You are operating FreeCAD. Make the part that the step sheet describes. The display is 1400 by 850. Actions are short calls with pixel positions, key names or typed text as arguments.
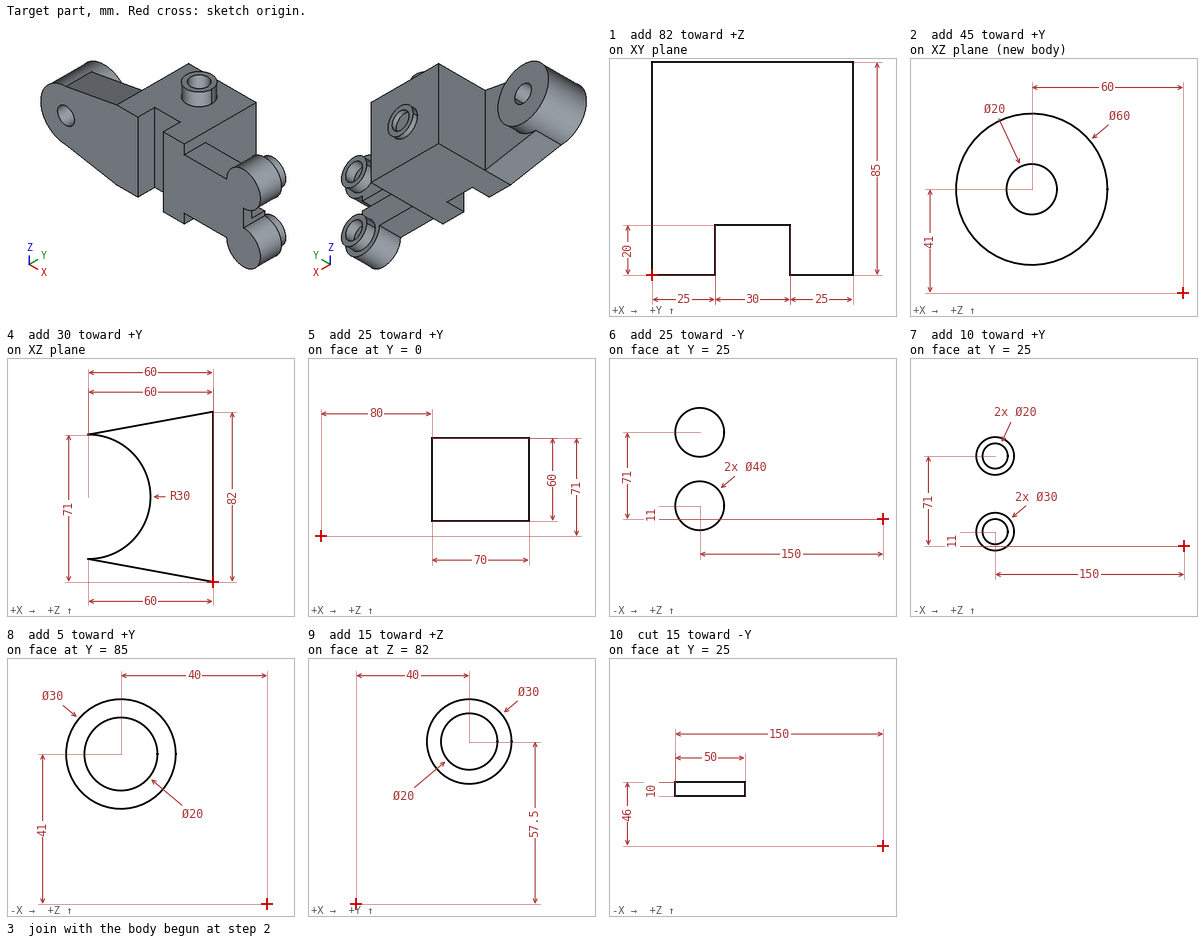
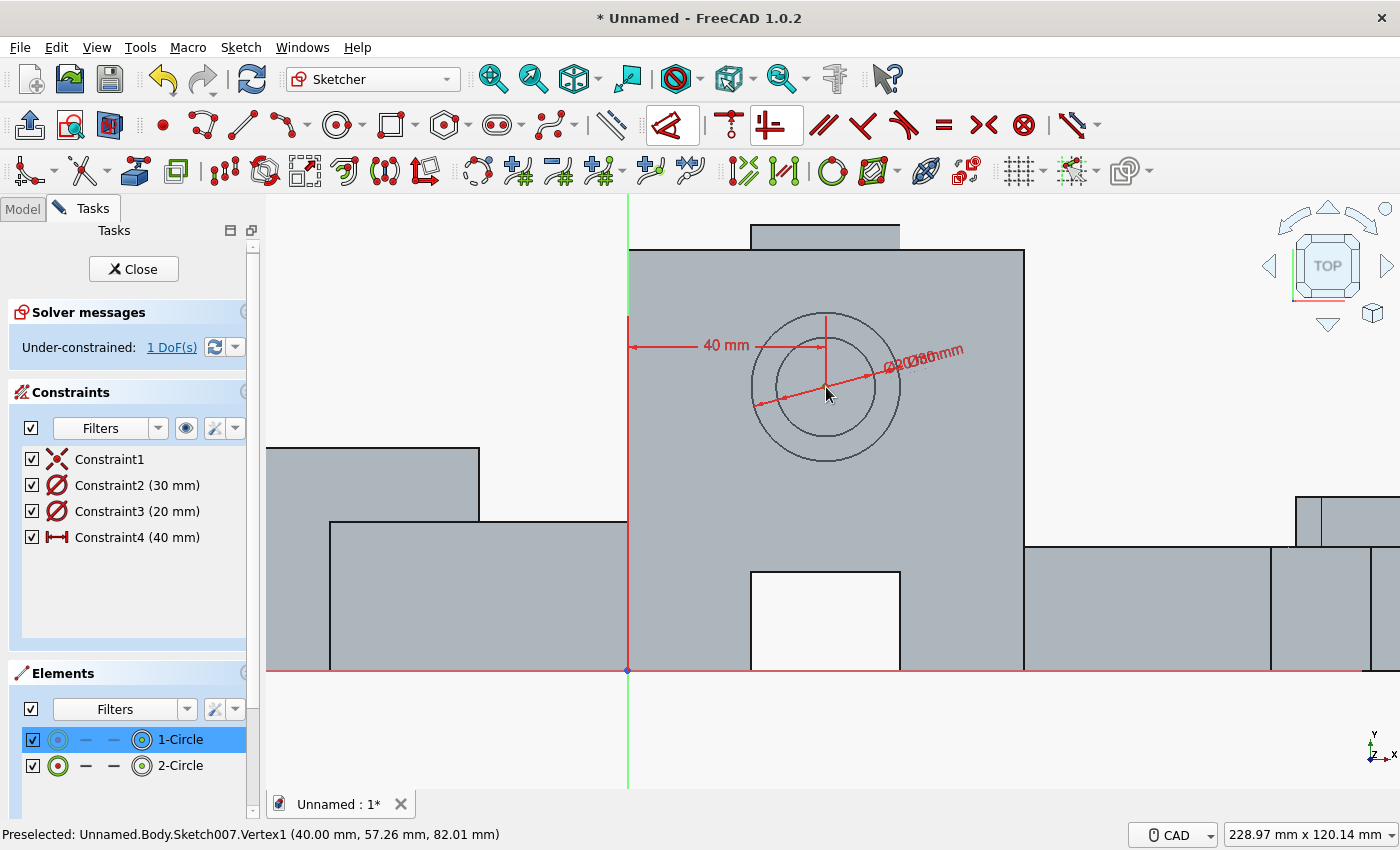
key(i)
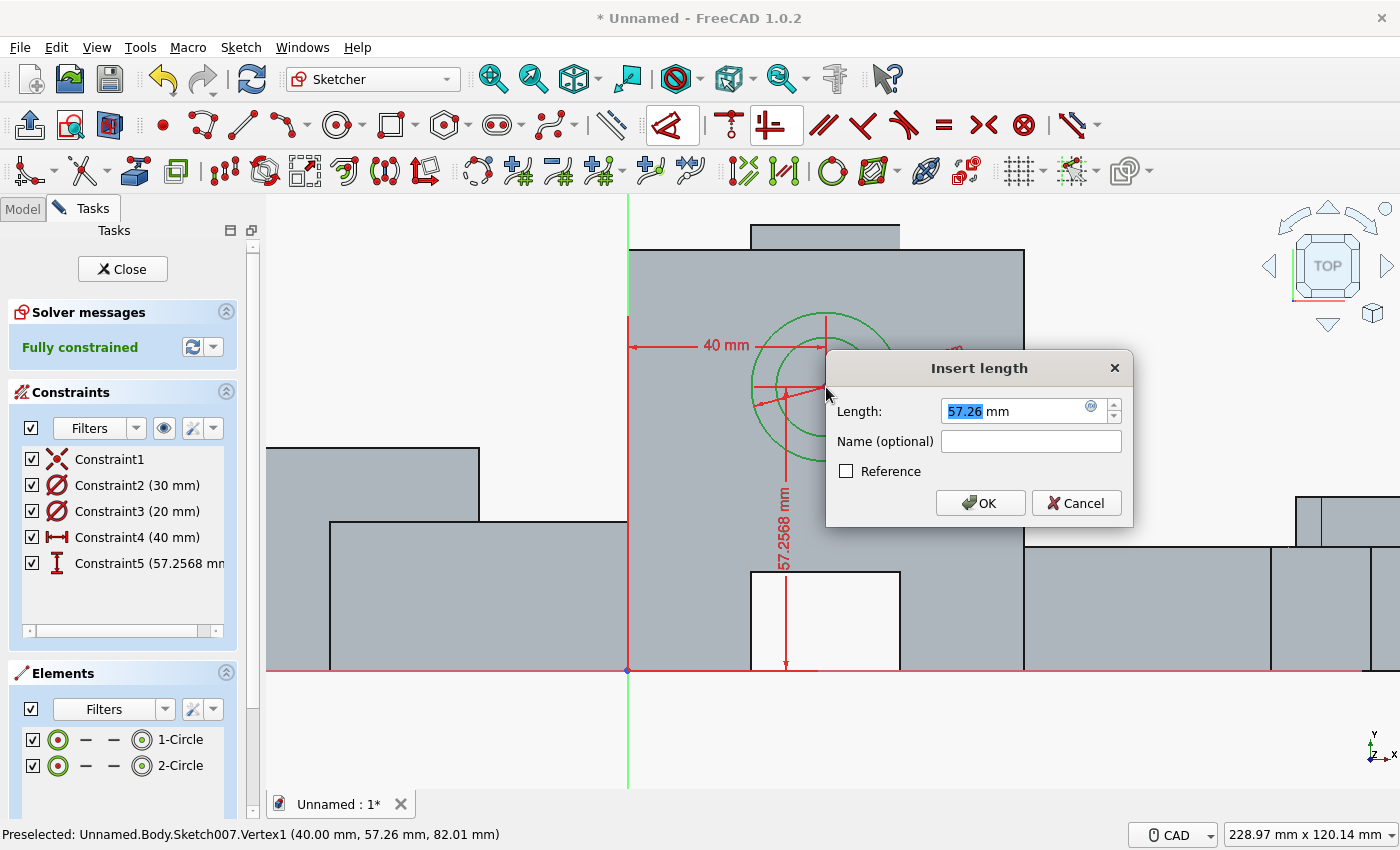
text(57.5)
key(Return)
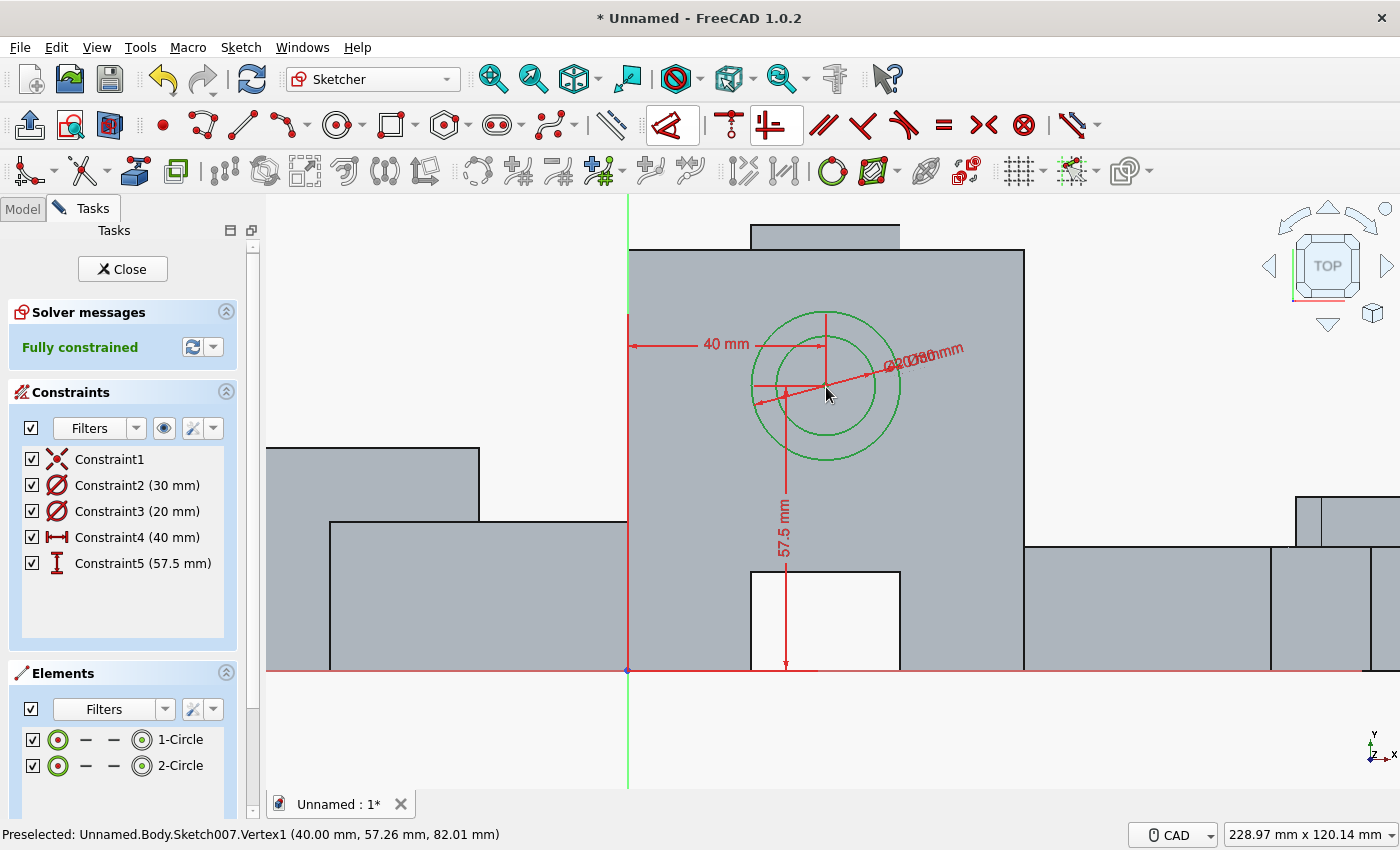
click(123, 269)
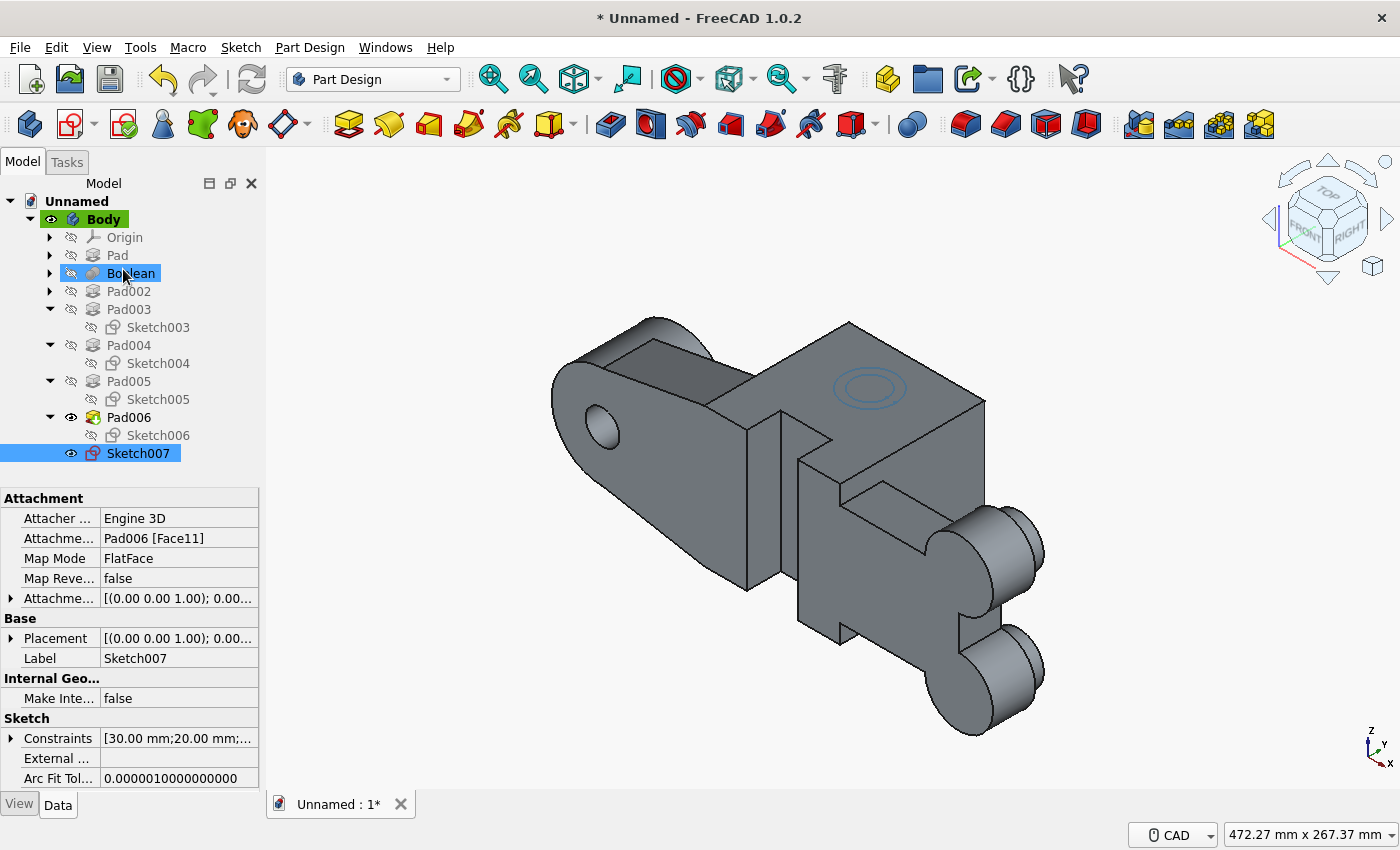
click(350, 124)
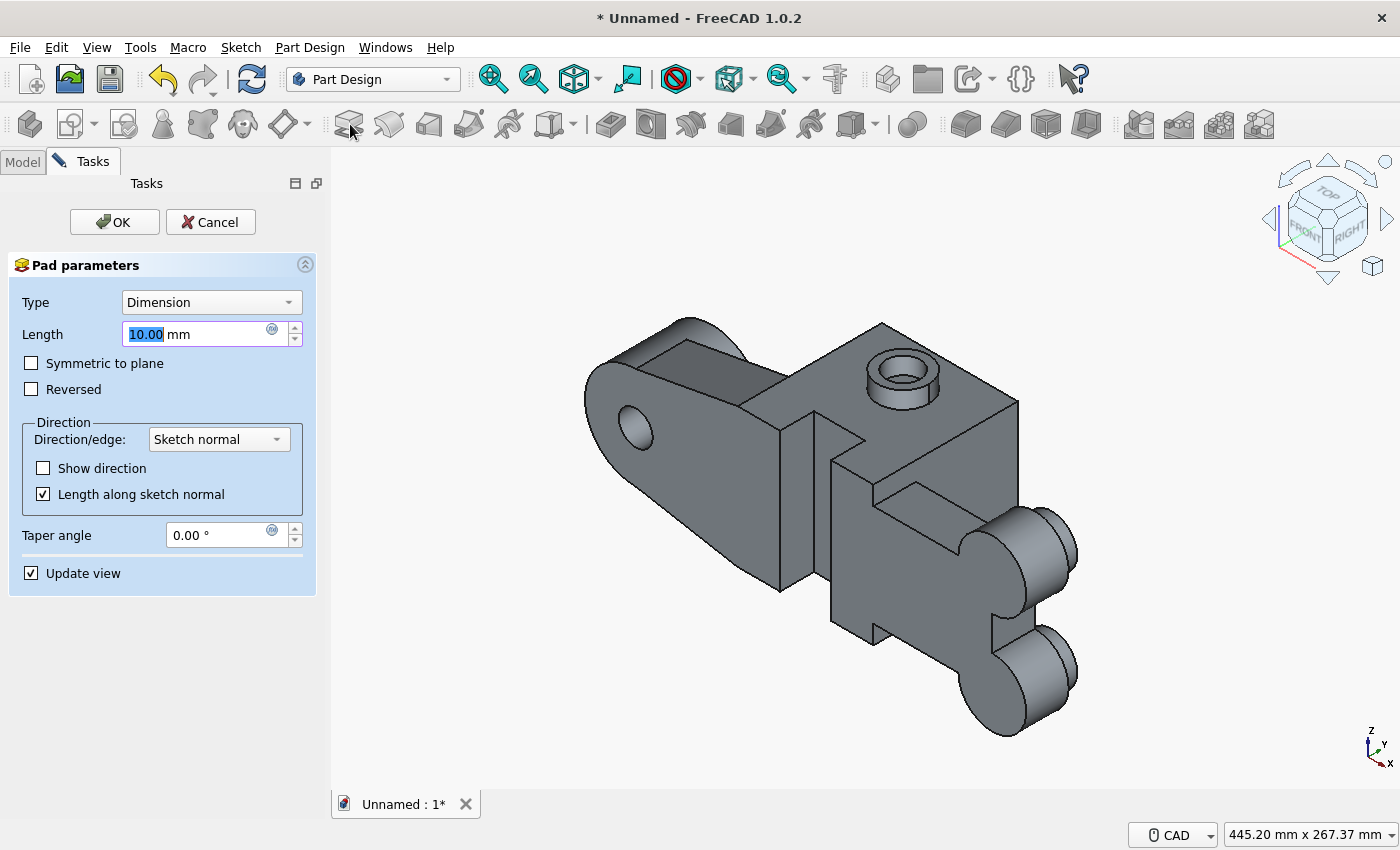
text(15)
key(Tab)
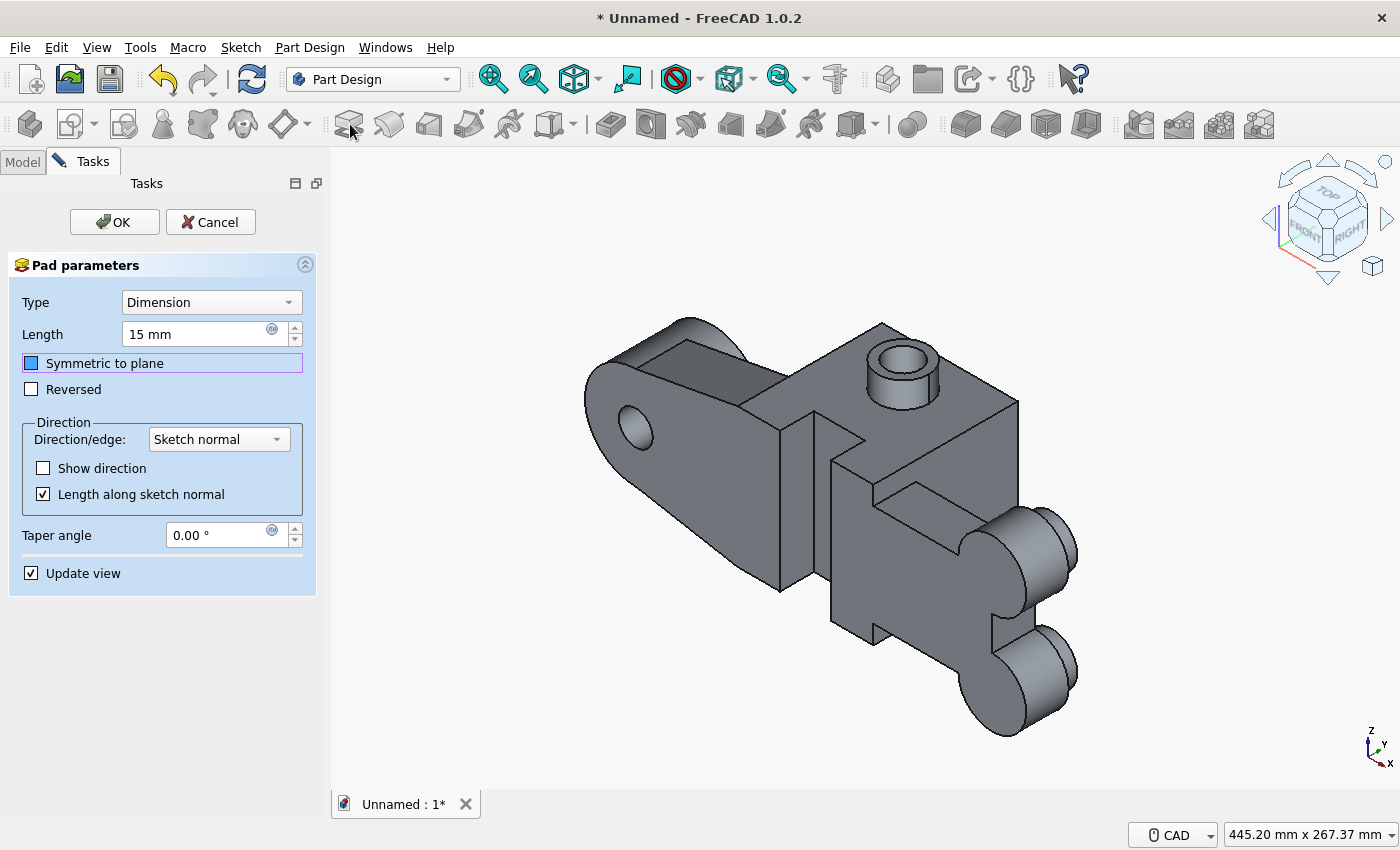
click(115, 222)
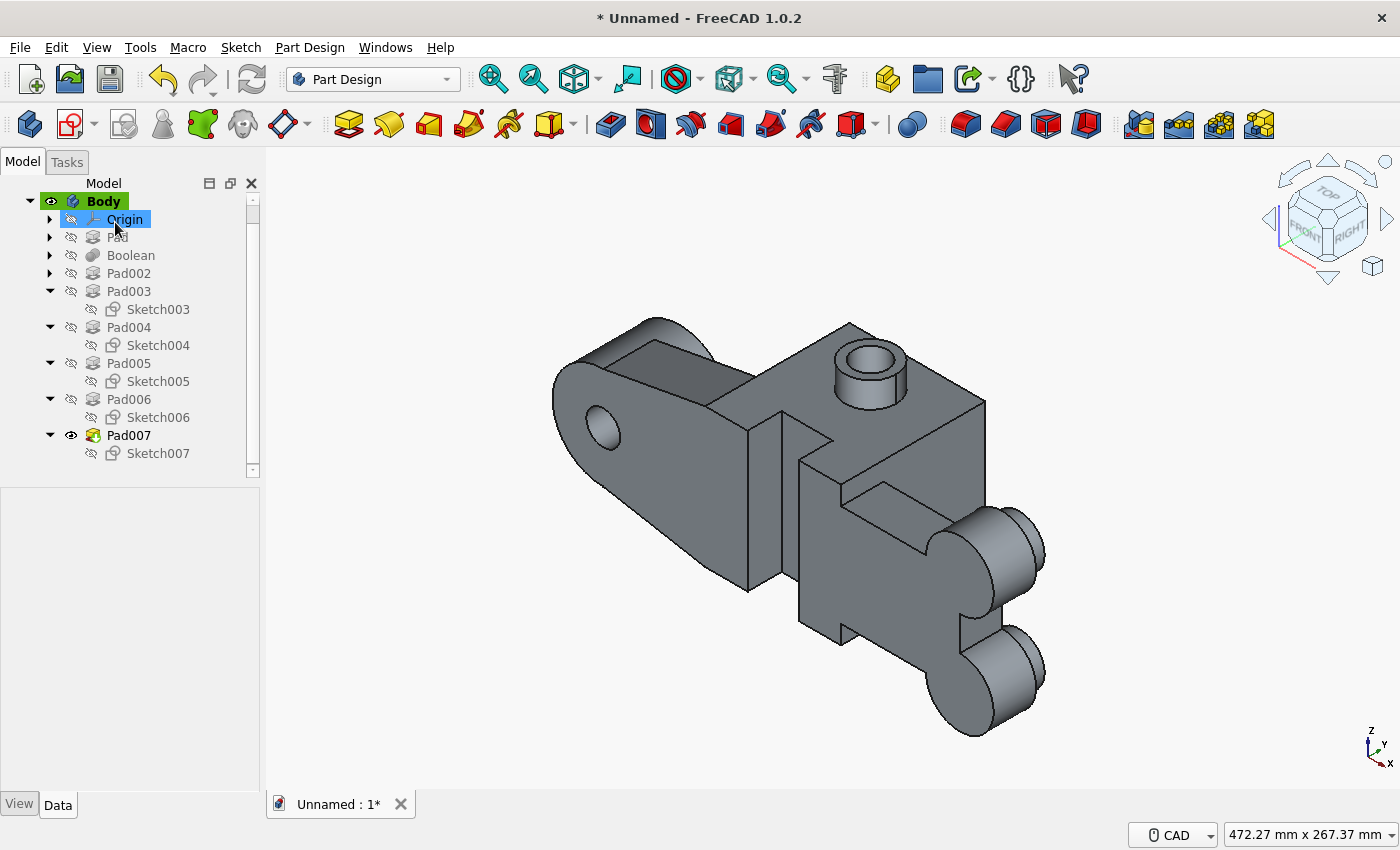
key(4)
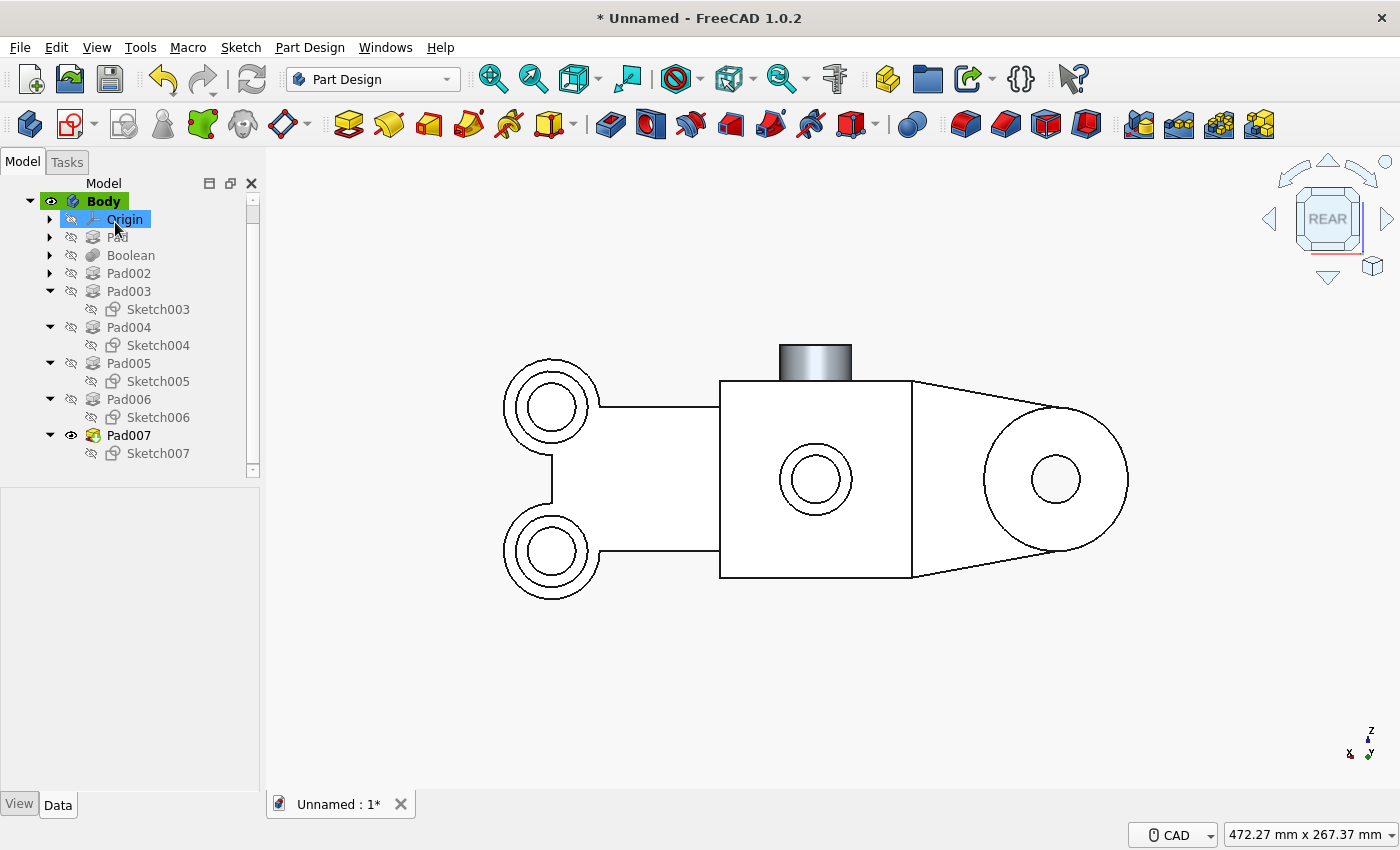
click(643, 478)